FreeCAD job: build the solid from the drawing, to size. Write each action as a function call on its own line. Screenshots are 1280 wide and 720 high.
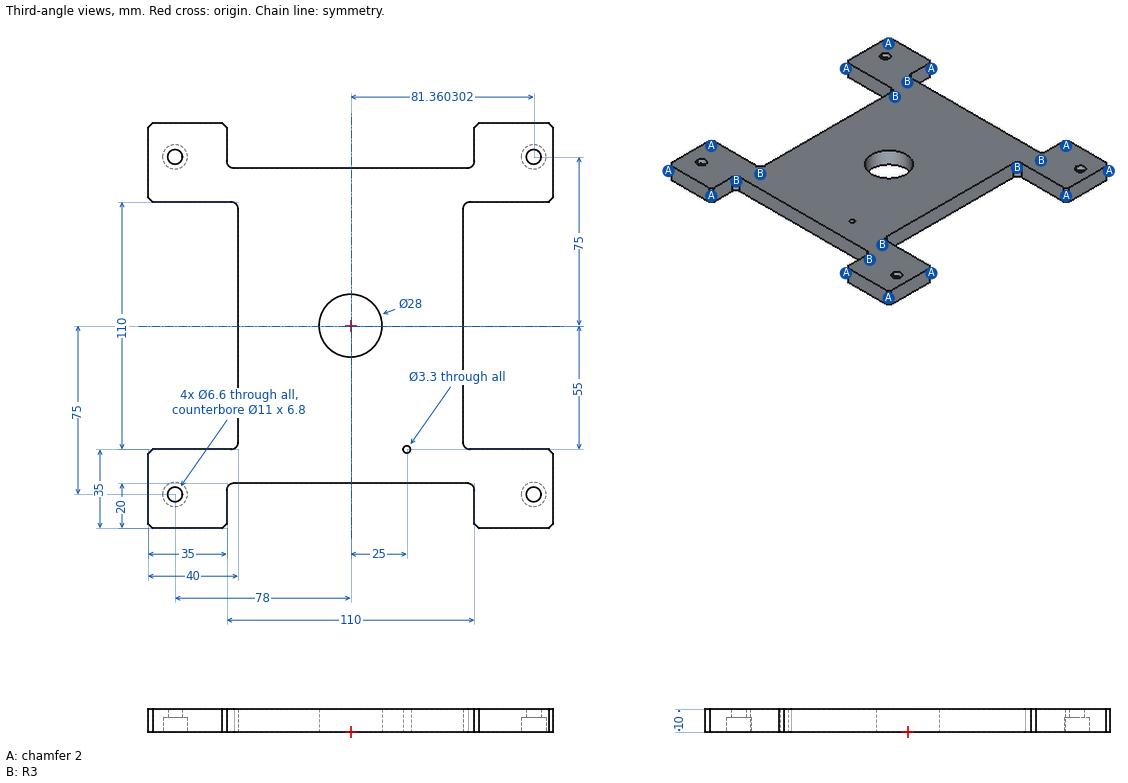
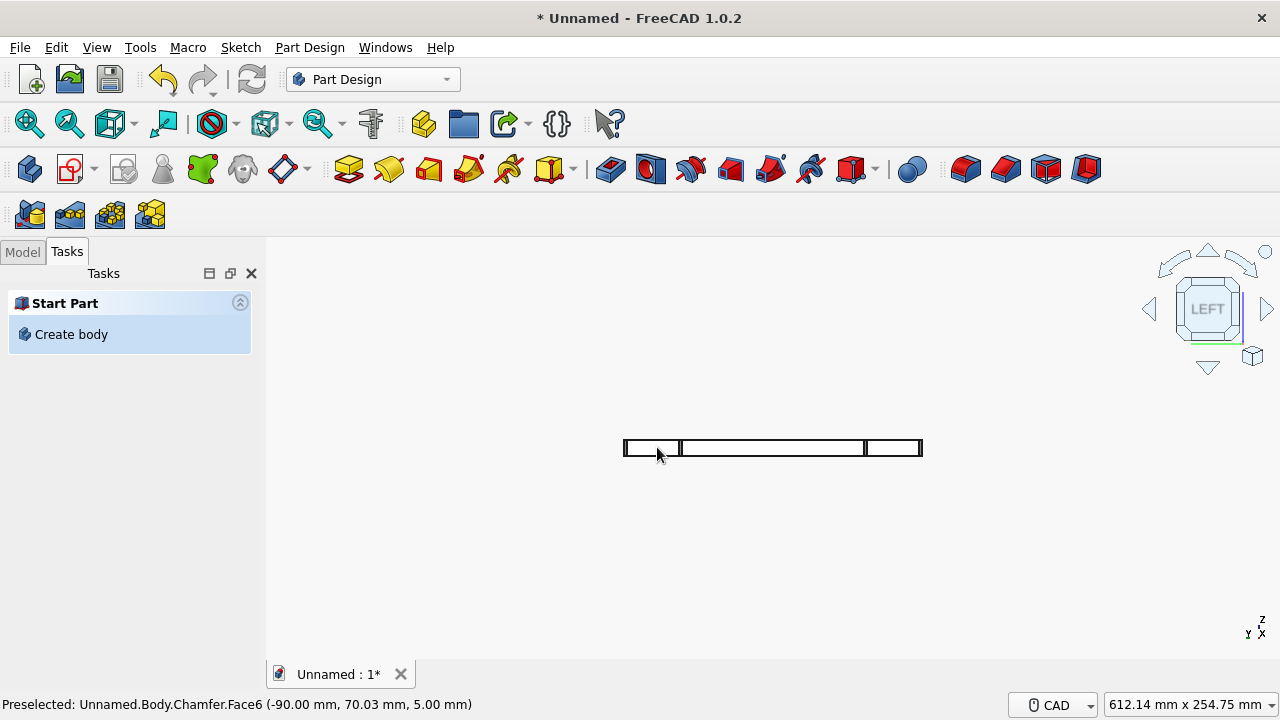
key(v)
key(3)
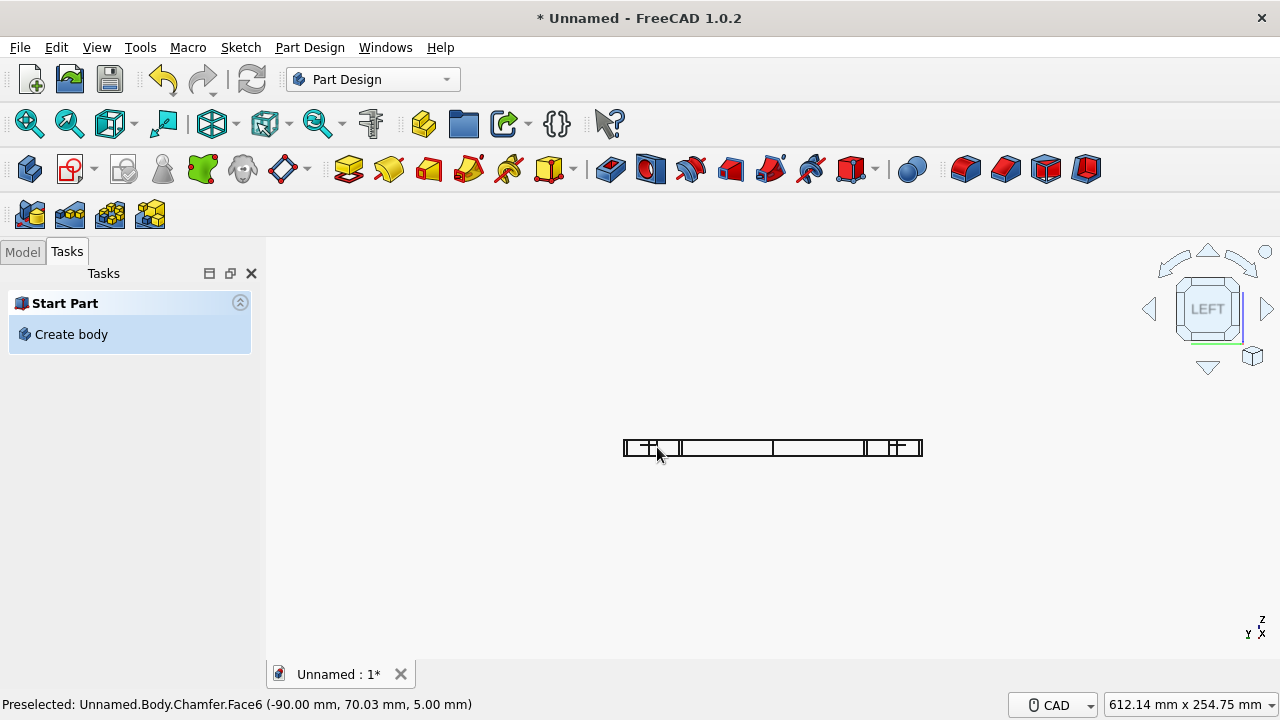
key(0)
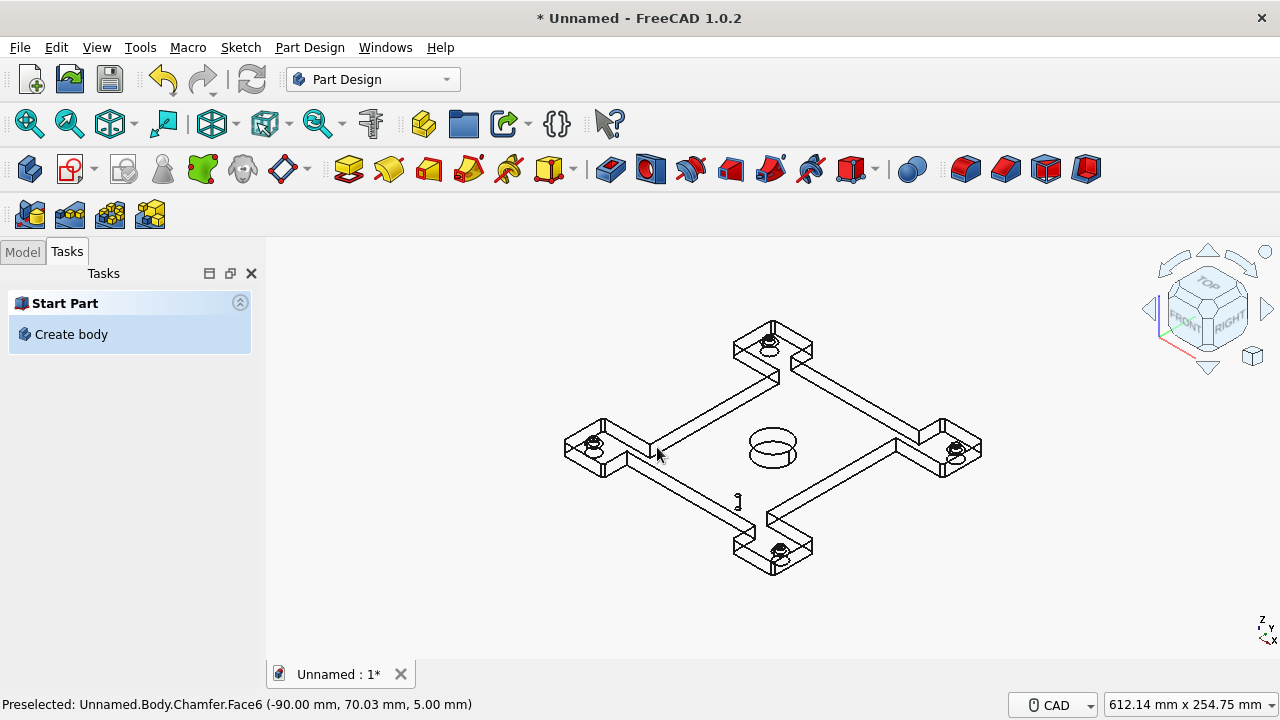
click(791, 364)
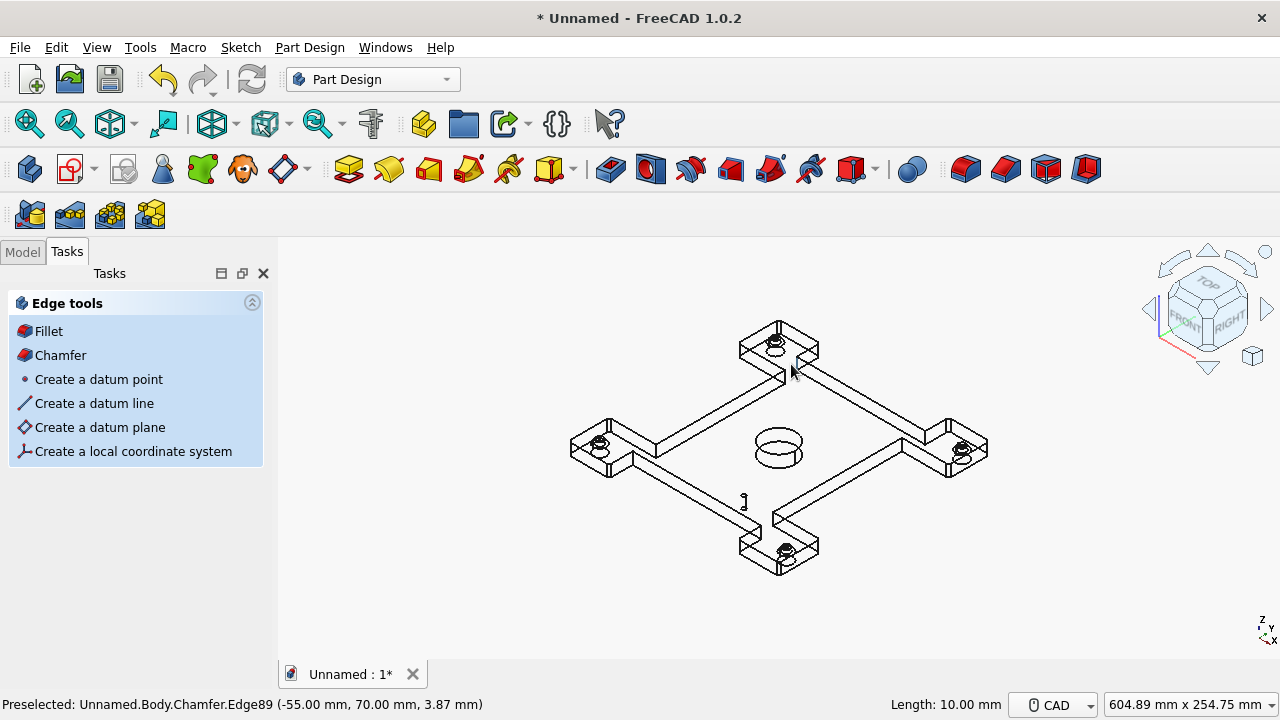
click(925, 437, ctrl)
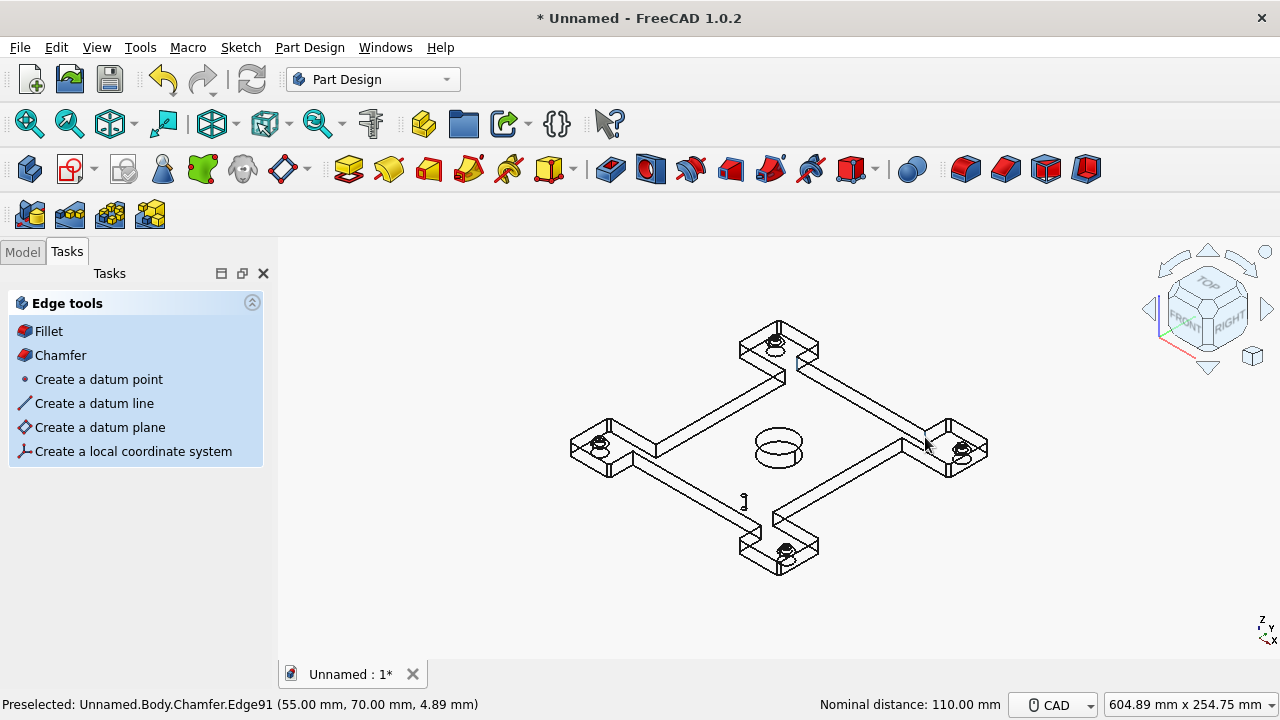
click(902, 445, ctrl)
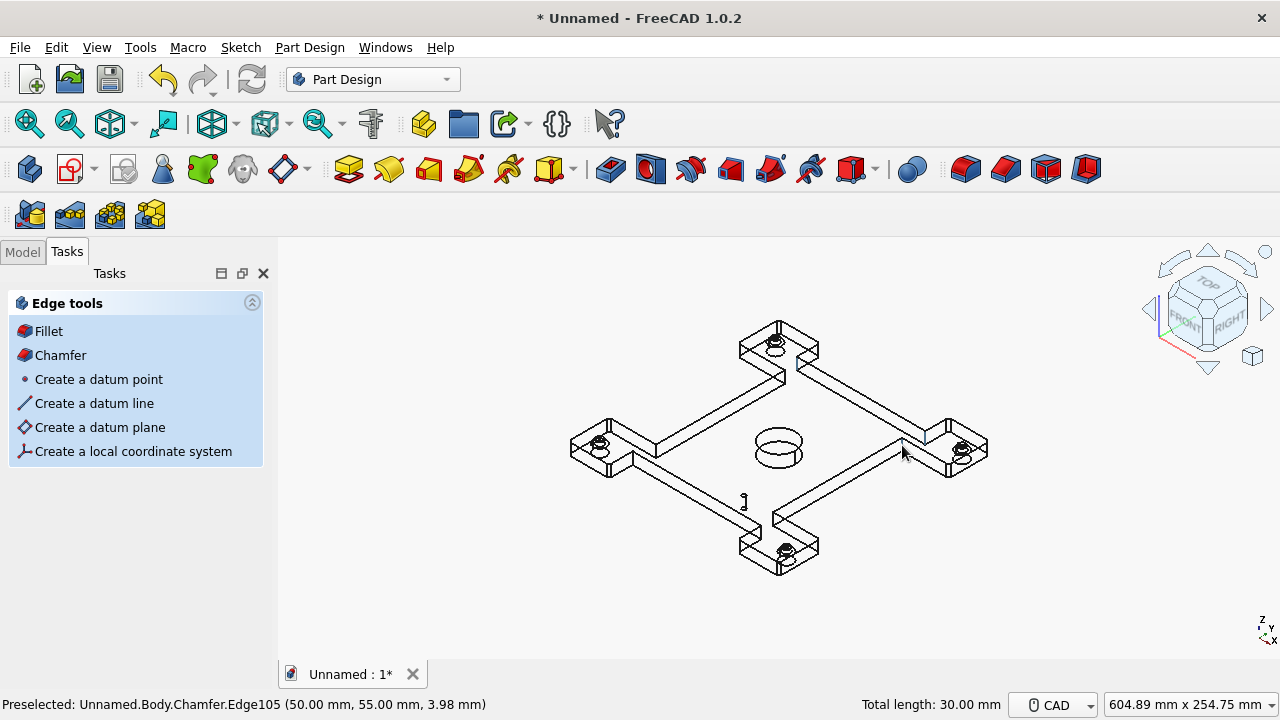
click(773, 519, ctrl)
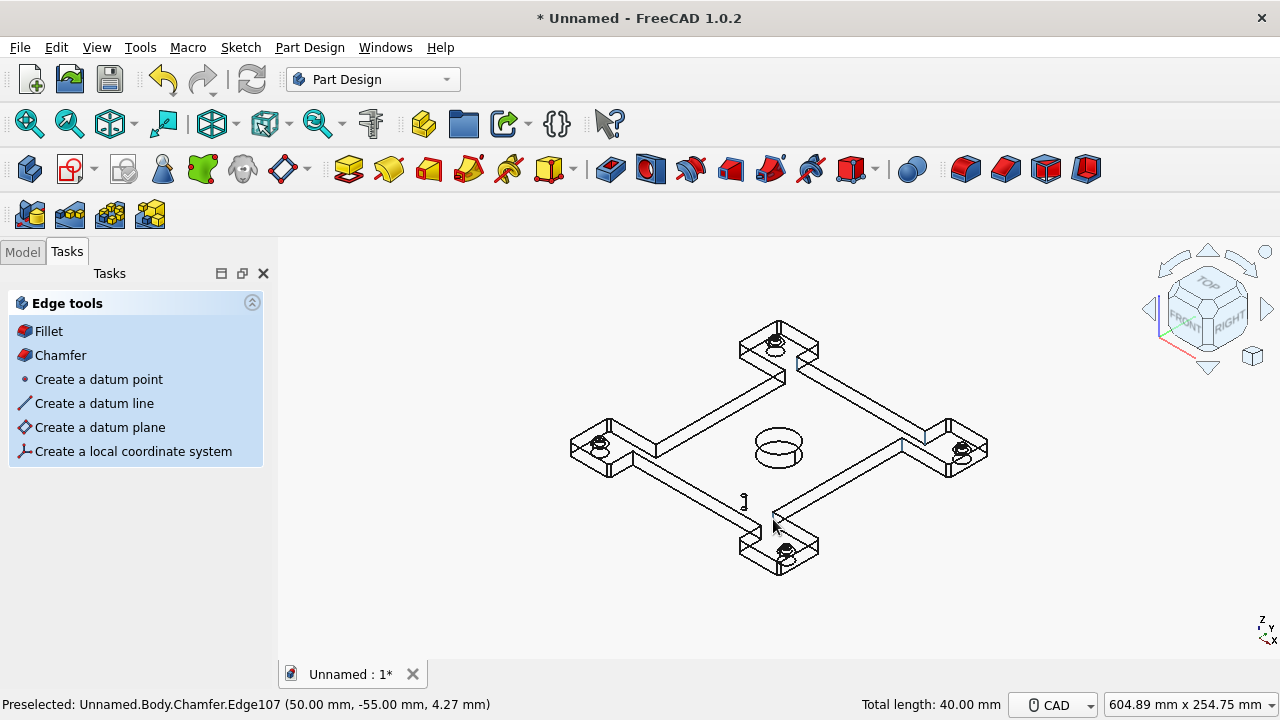
click(761, 533, ctrl)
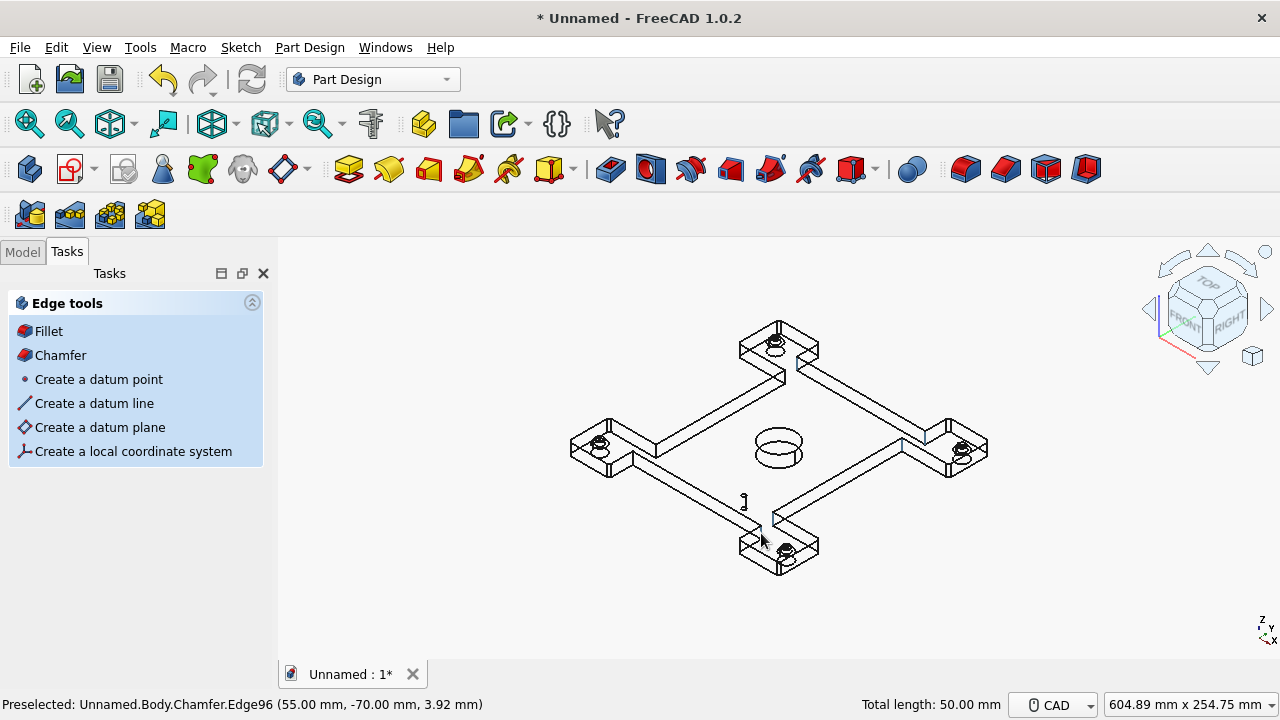
click(633, 458, ctrl)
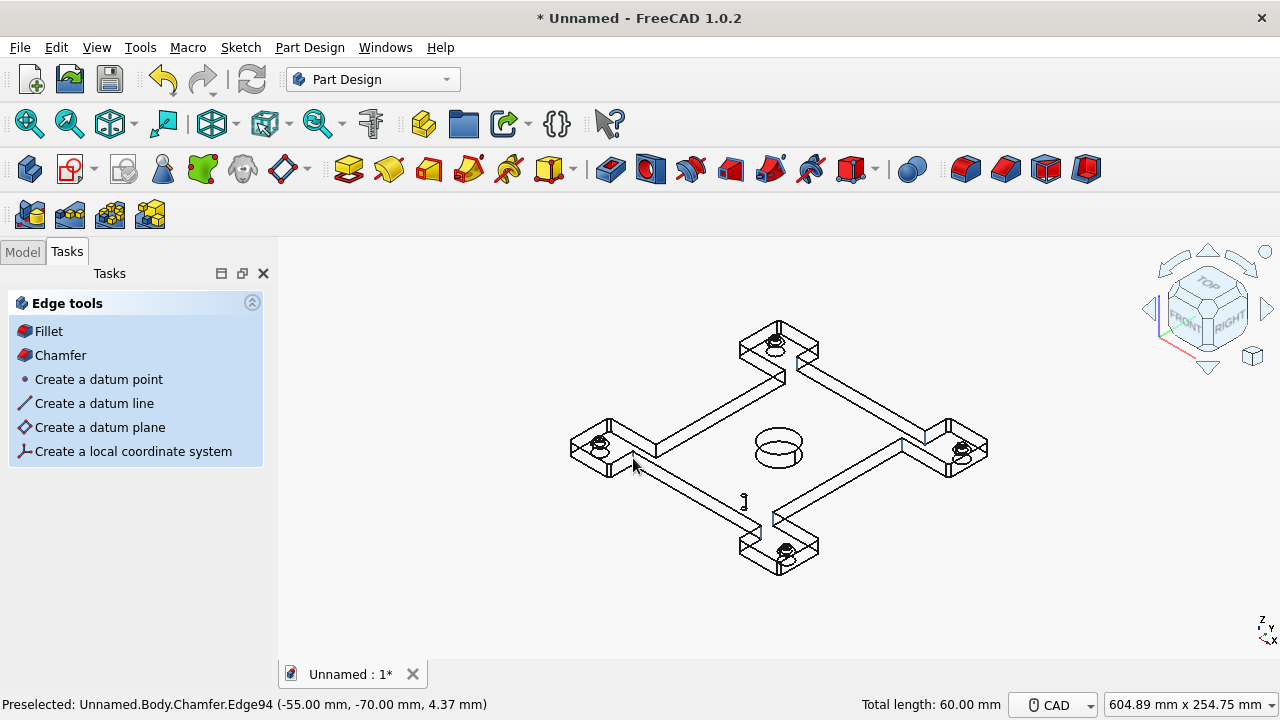
click(656, 450, ctrl)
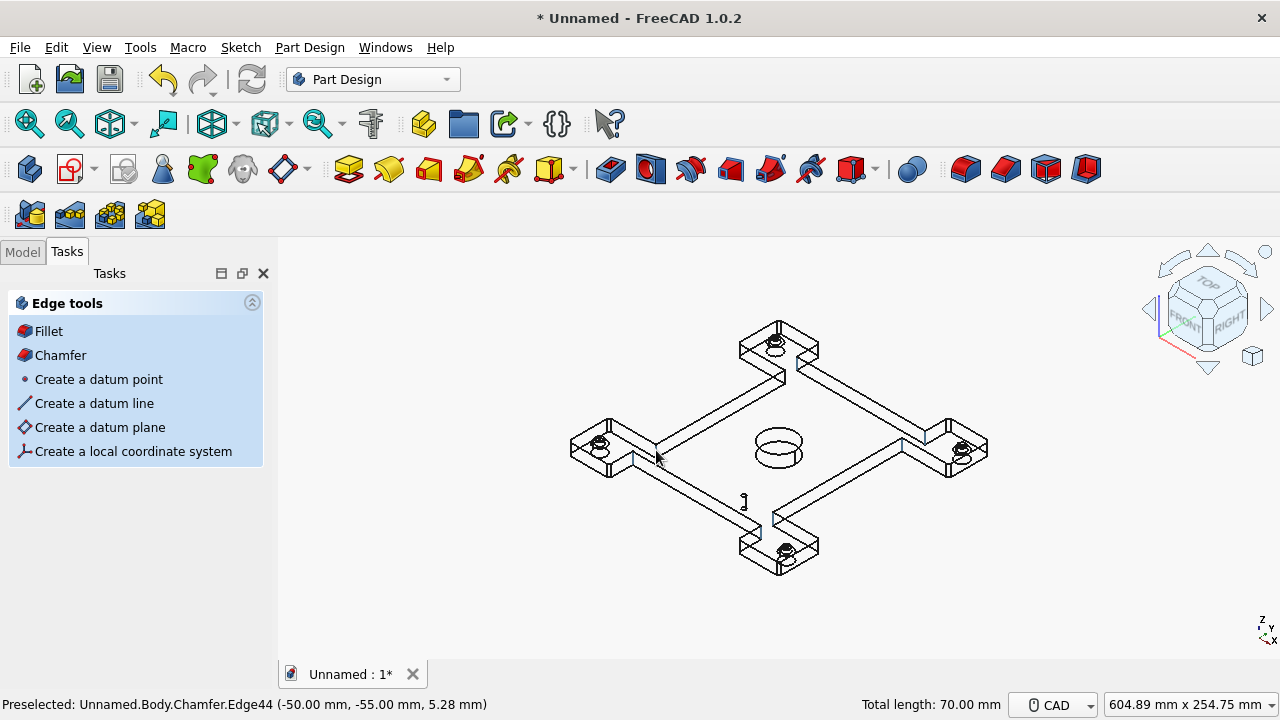
click(785, 377, ctrl)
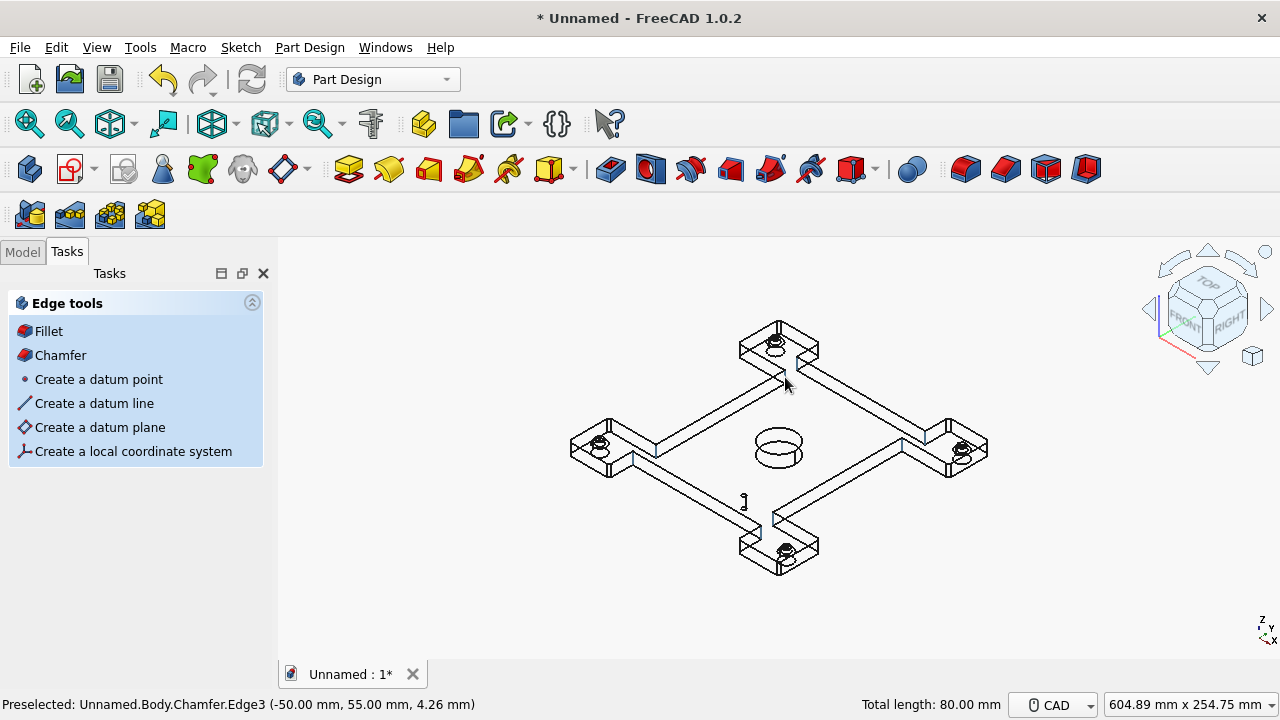
key(v)
key(1)